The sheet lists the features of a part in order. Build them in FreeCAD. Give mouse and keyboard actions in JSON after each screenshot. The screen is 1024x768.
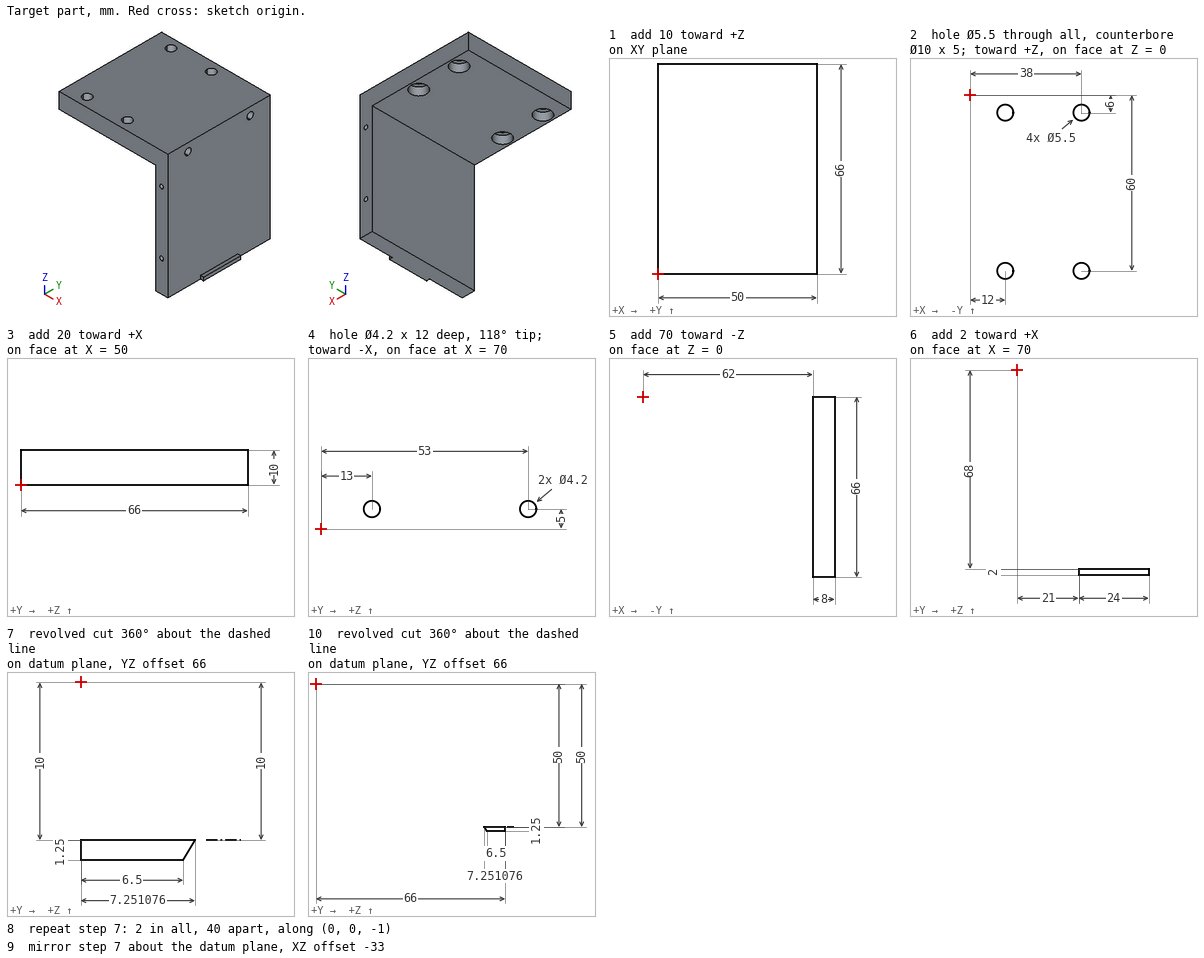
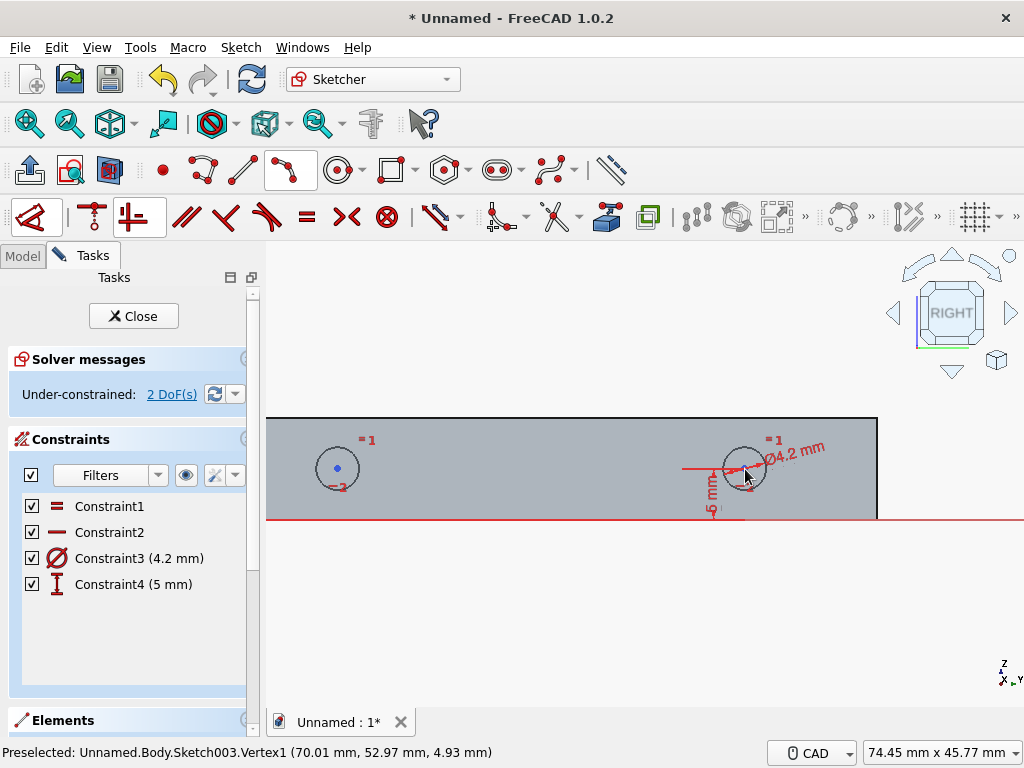
{"action": "left_click", "coordinate": [745, 469]}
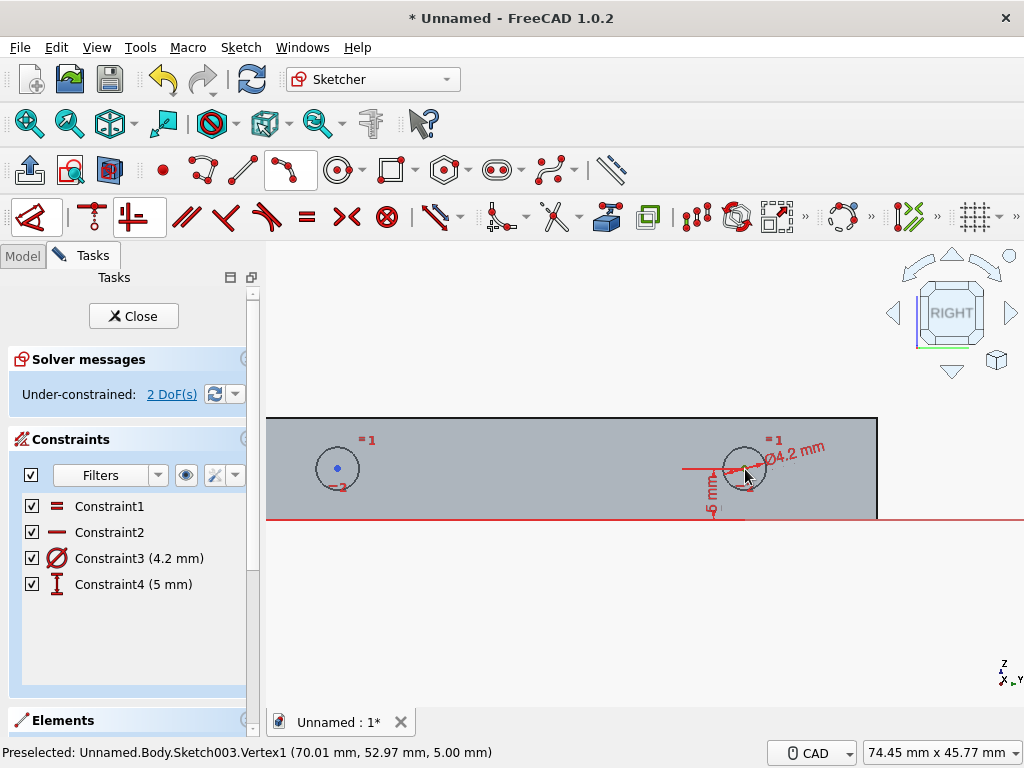
{"action": "left_click", "coordinate": [56, 218]}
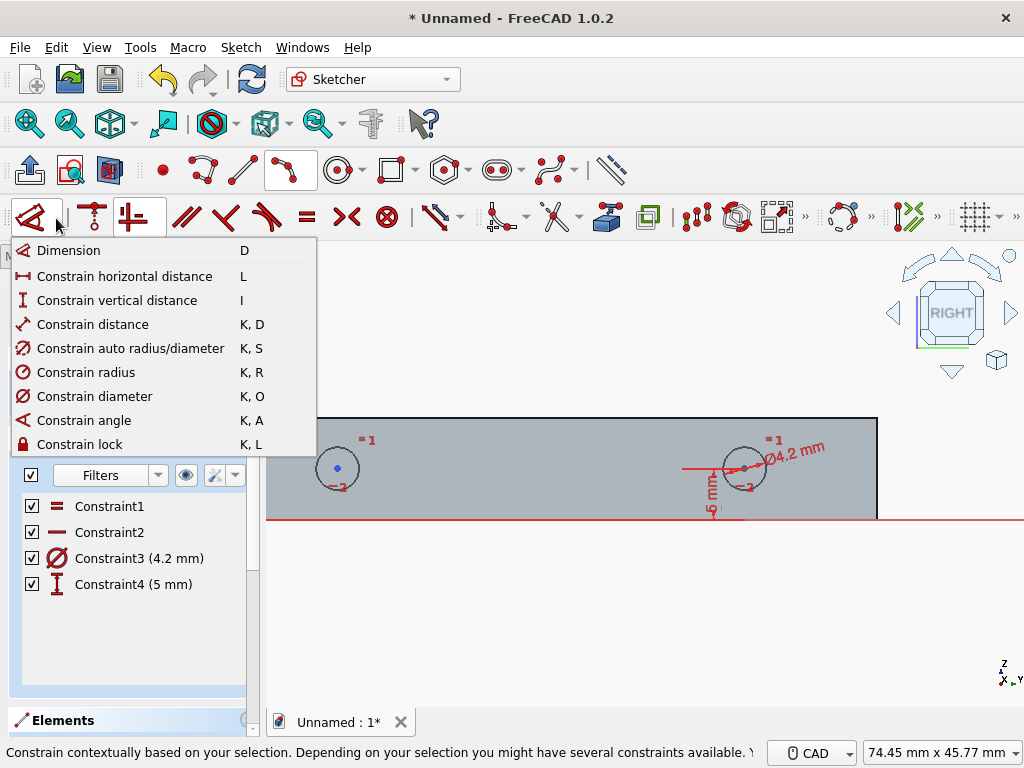
{"action": "left_click", "coordinate": [164, 276]}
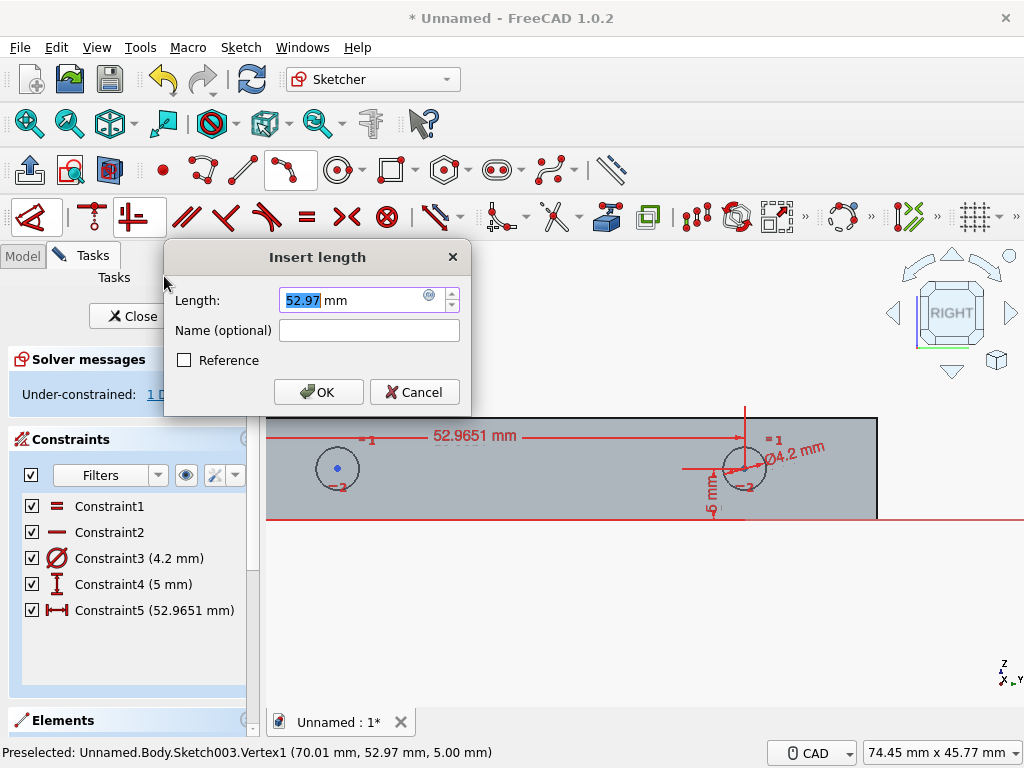
{"action": "type", "text": "53"}
{"action": "key", "text": "Return"}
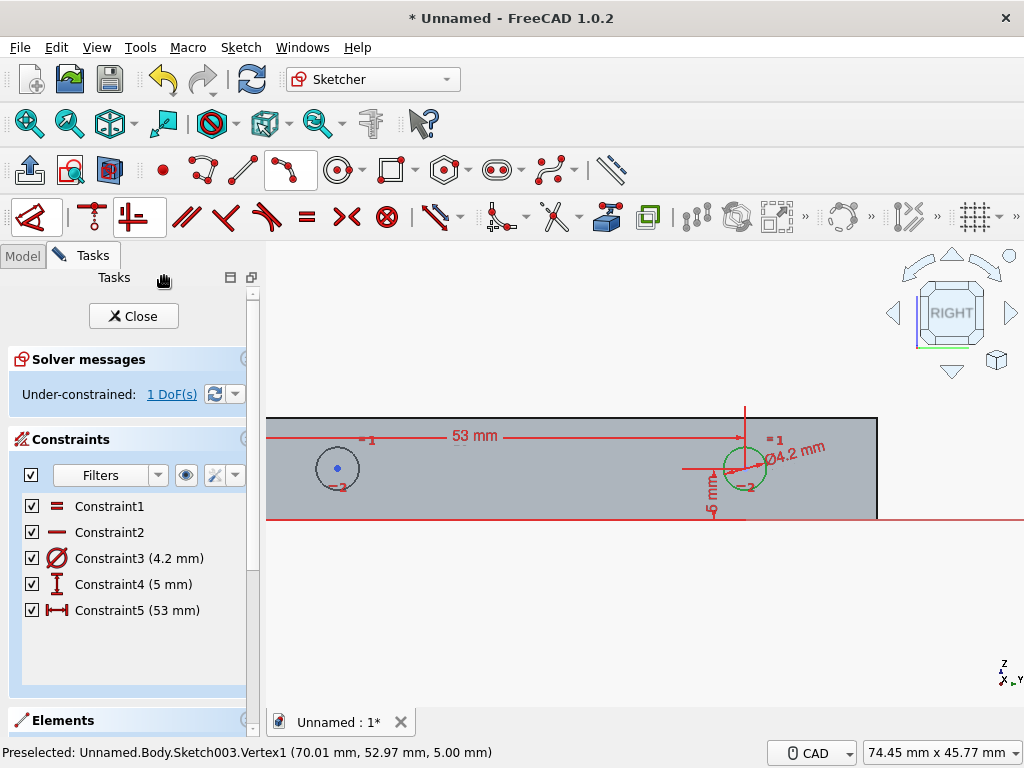
{"action": "left_click", "coordinate": [338, 469]}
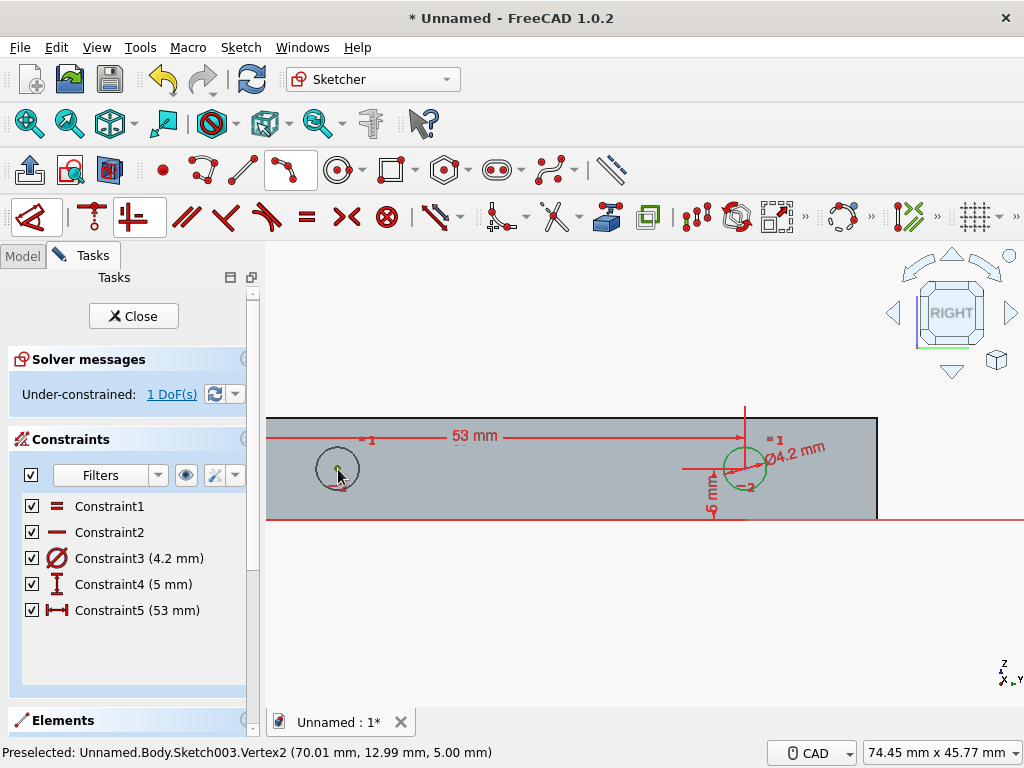
{"action": "key", "text": "l"}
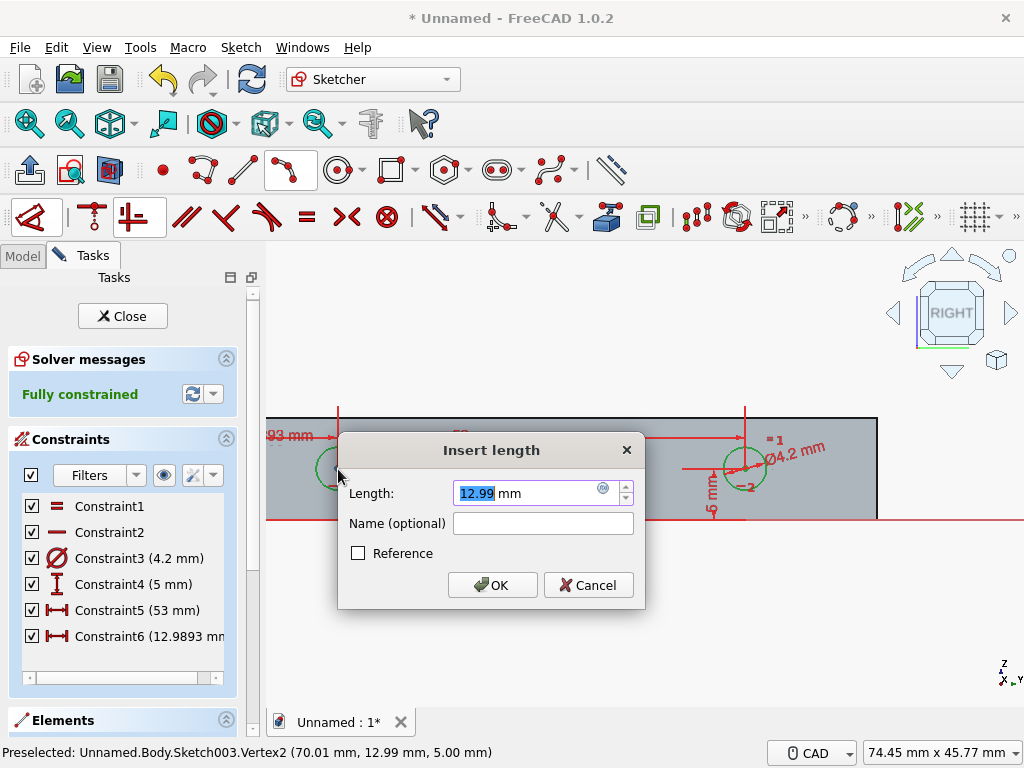
{"action": "type", "text": "13"}
{"action": "key", "text": "Return"}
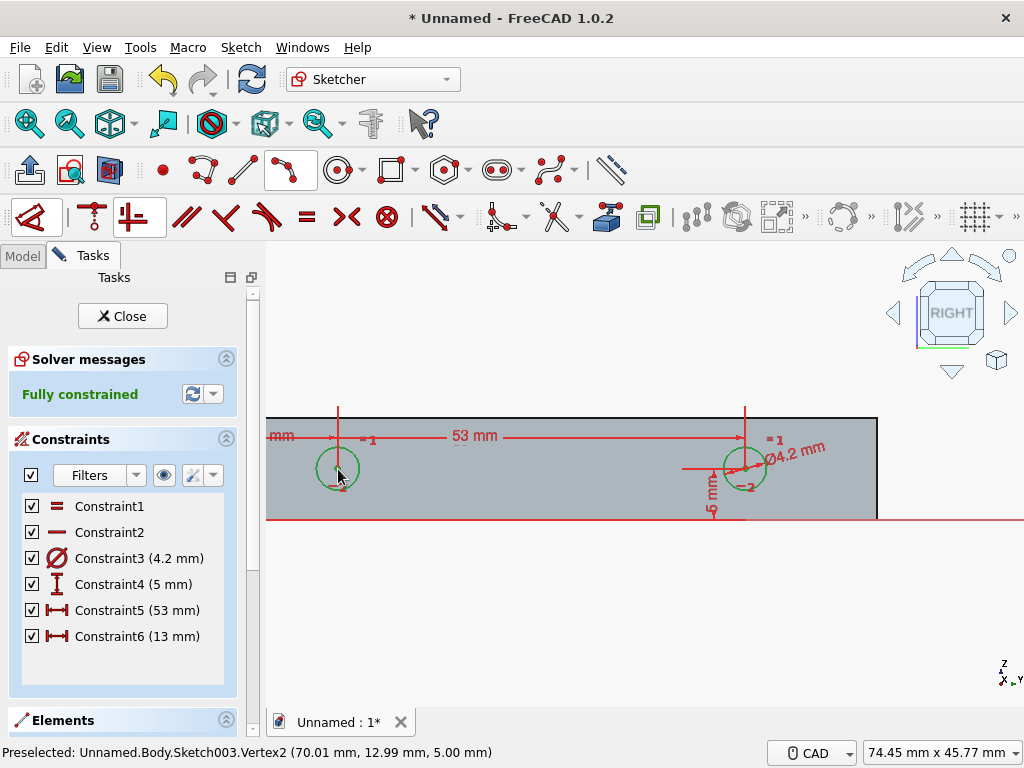
{"action": "left_click", "coordinate": [123, 316]}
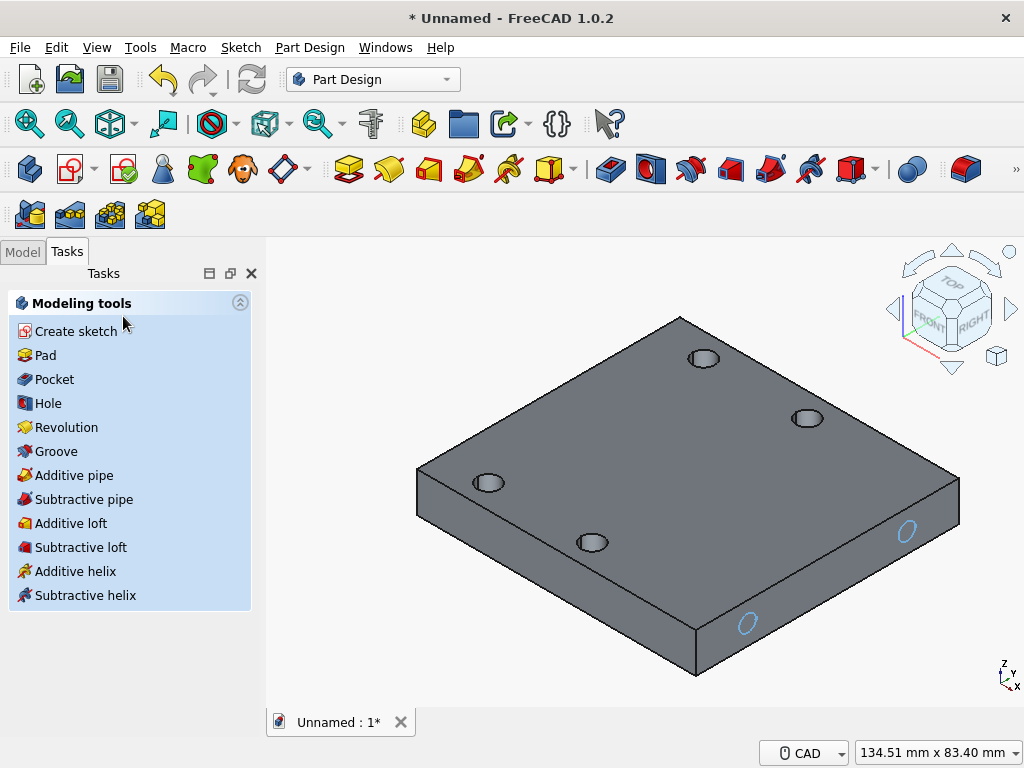
{"action": "left_click", "coordinate": [652, 170]}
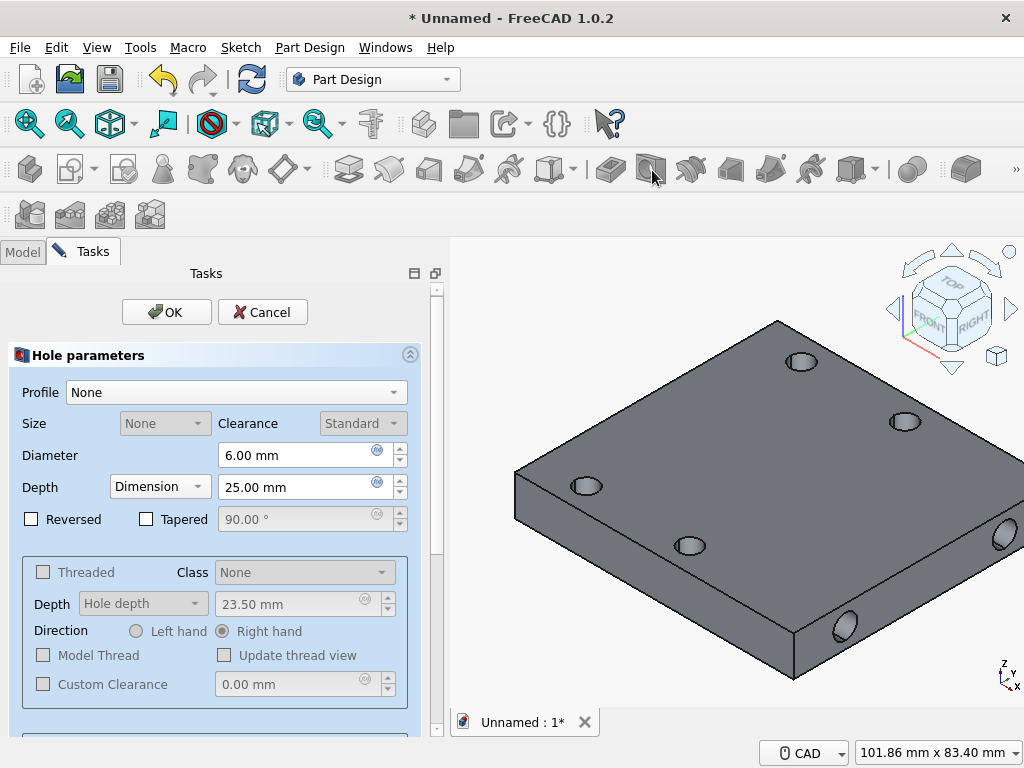
{"action": "triple_click", "coordinate": [305, 455]}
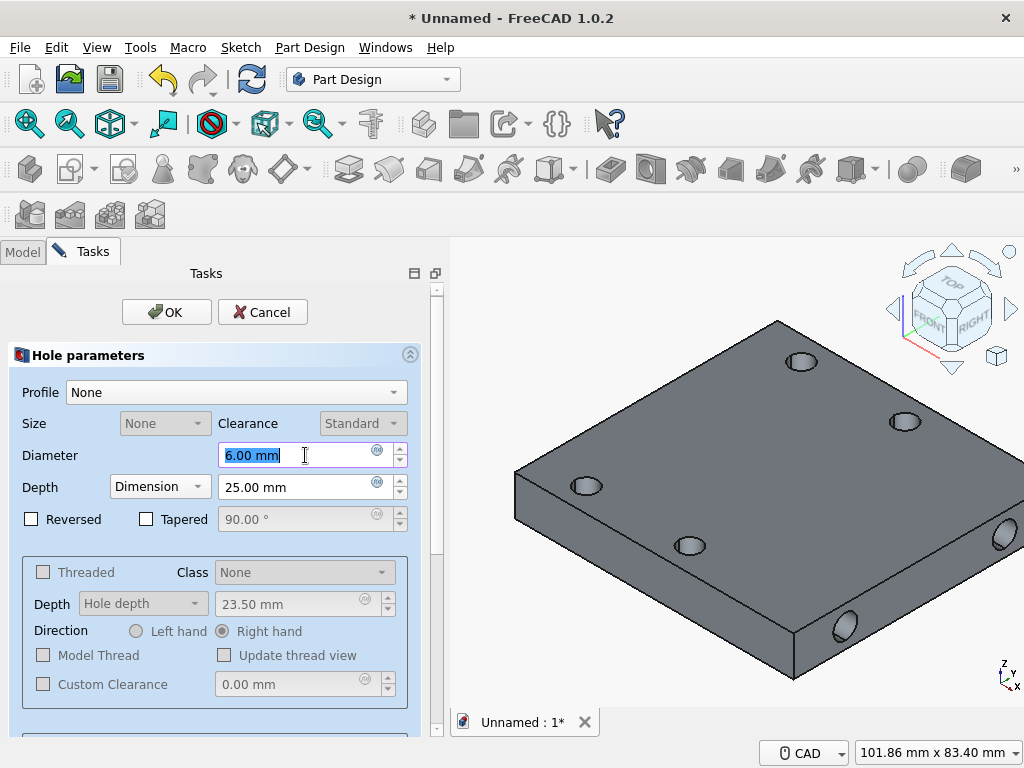
{"action": "type", "text": "4.2"}
{"action": "key", "text": "Tab"}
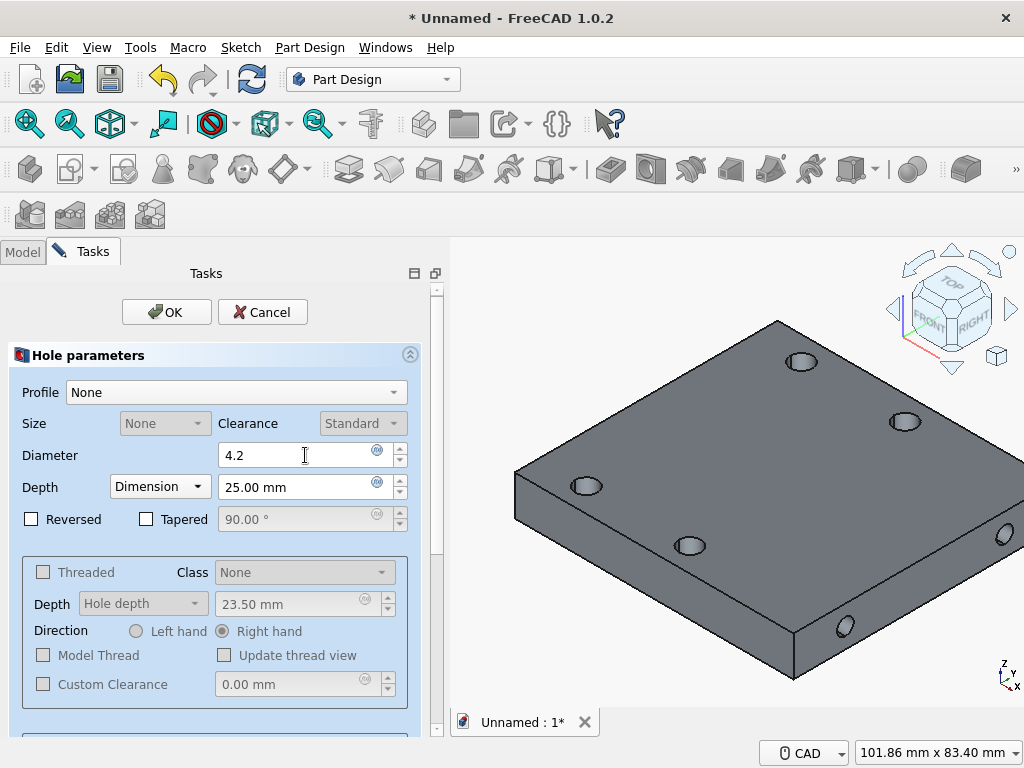
{"action": "triple_click", "coordinate": [305, 487]}